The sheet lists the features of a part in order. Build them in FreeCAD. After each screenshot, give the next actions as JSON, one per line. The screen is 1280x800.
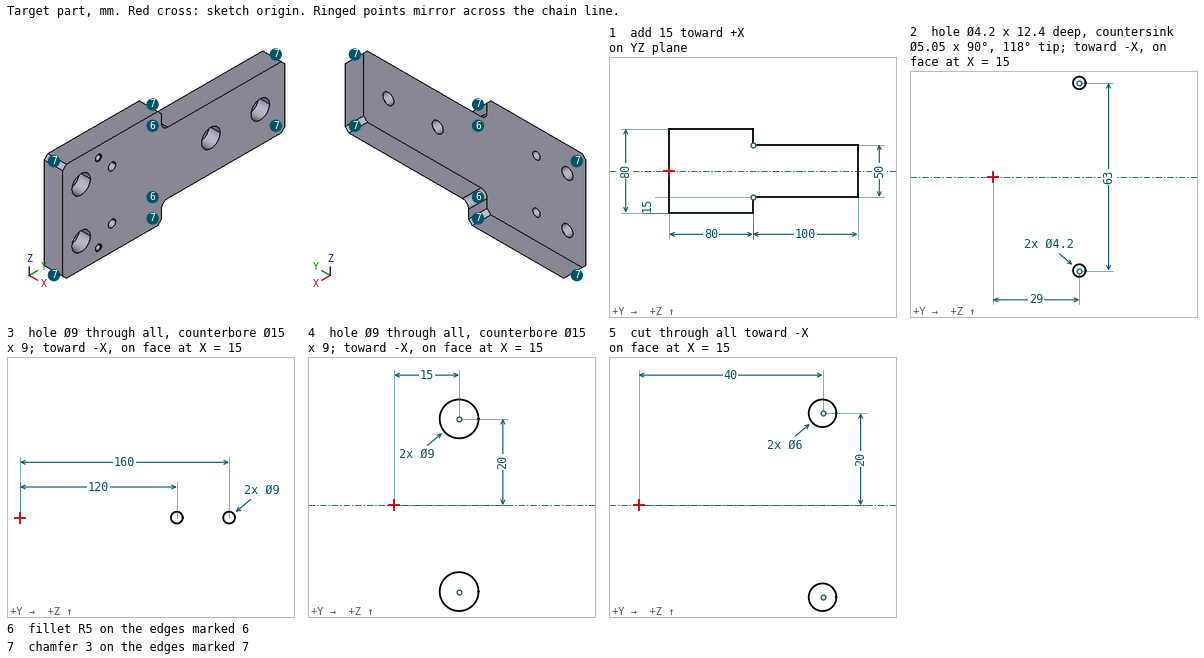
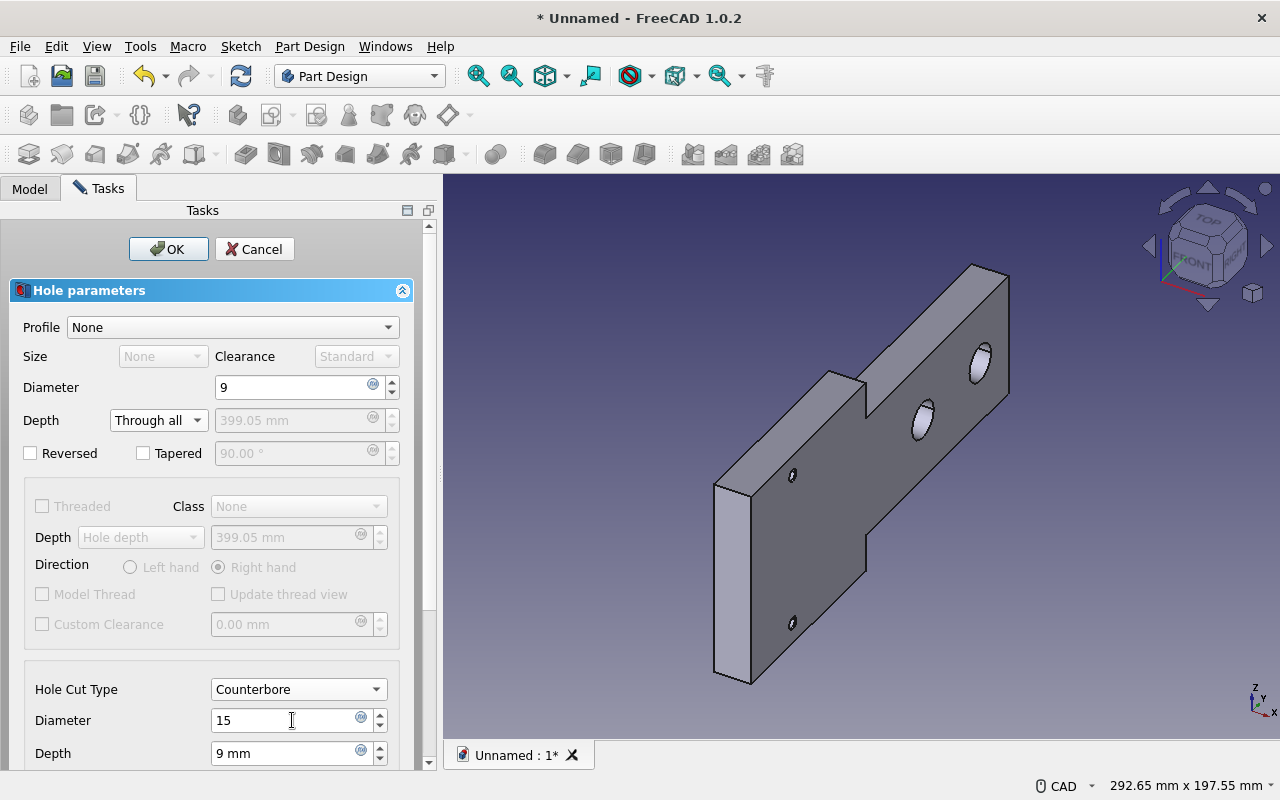
{"action": "left_click", "coordinate": [169, 249]}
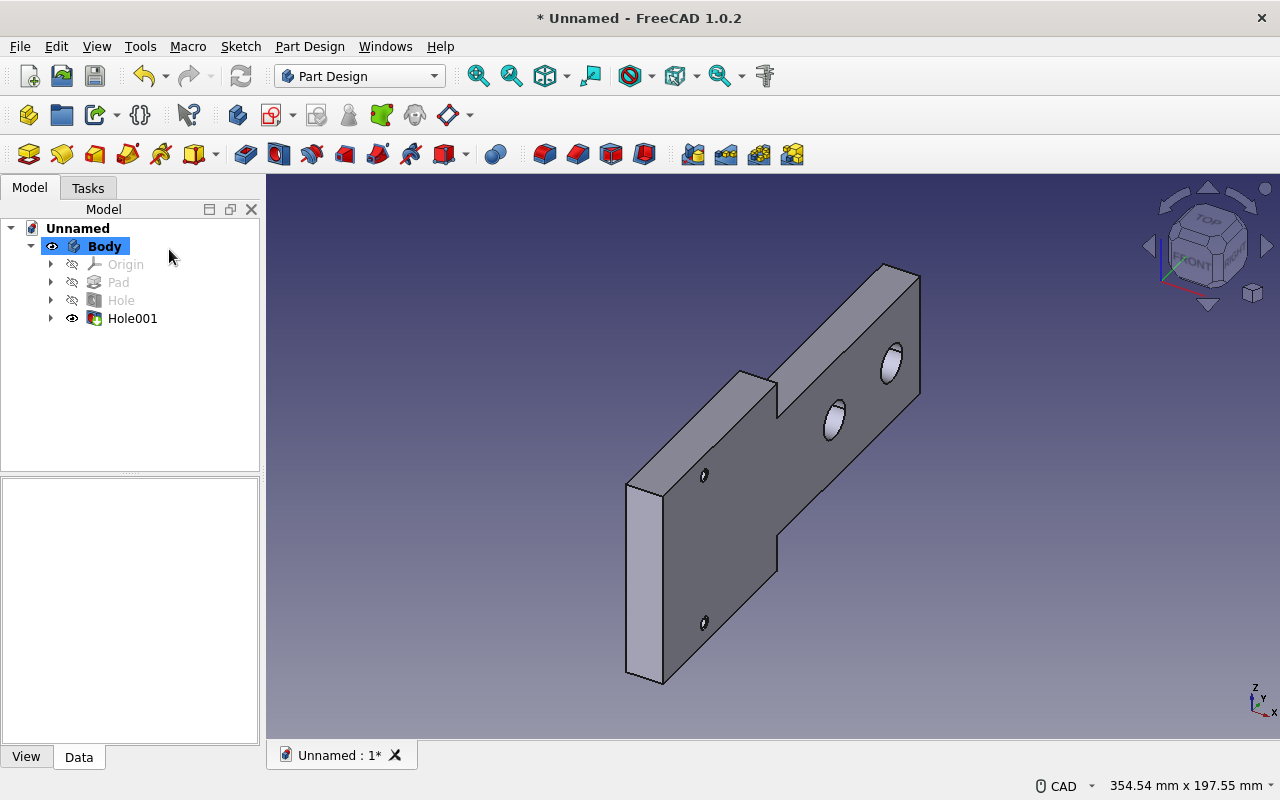
{"action": "left_click", "coordinate": [718, 535]}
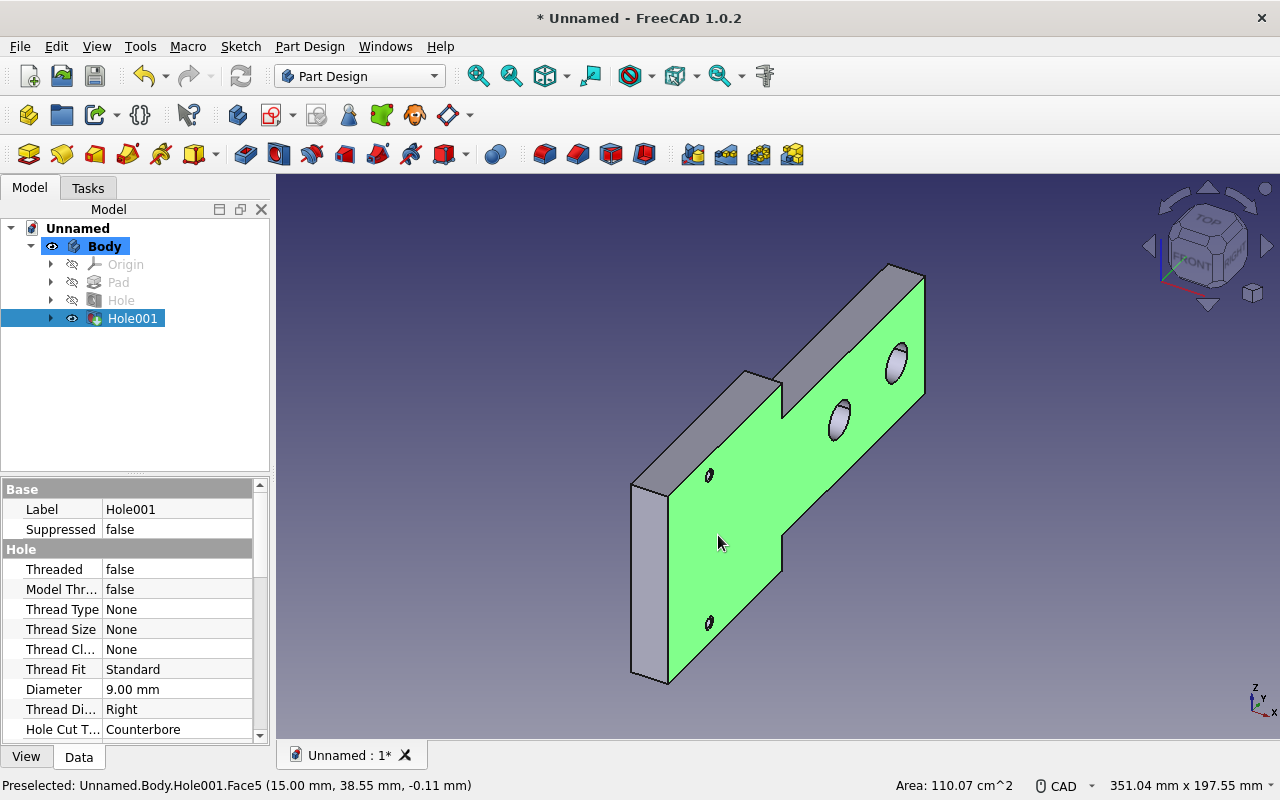
{"action": "left_click", "coordinate": [270, 116]}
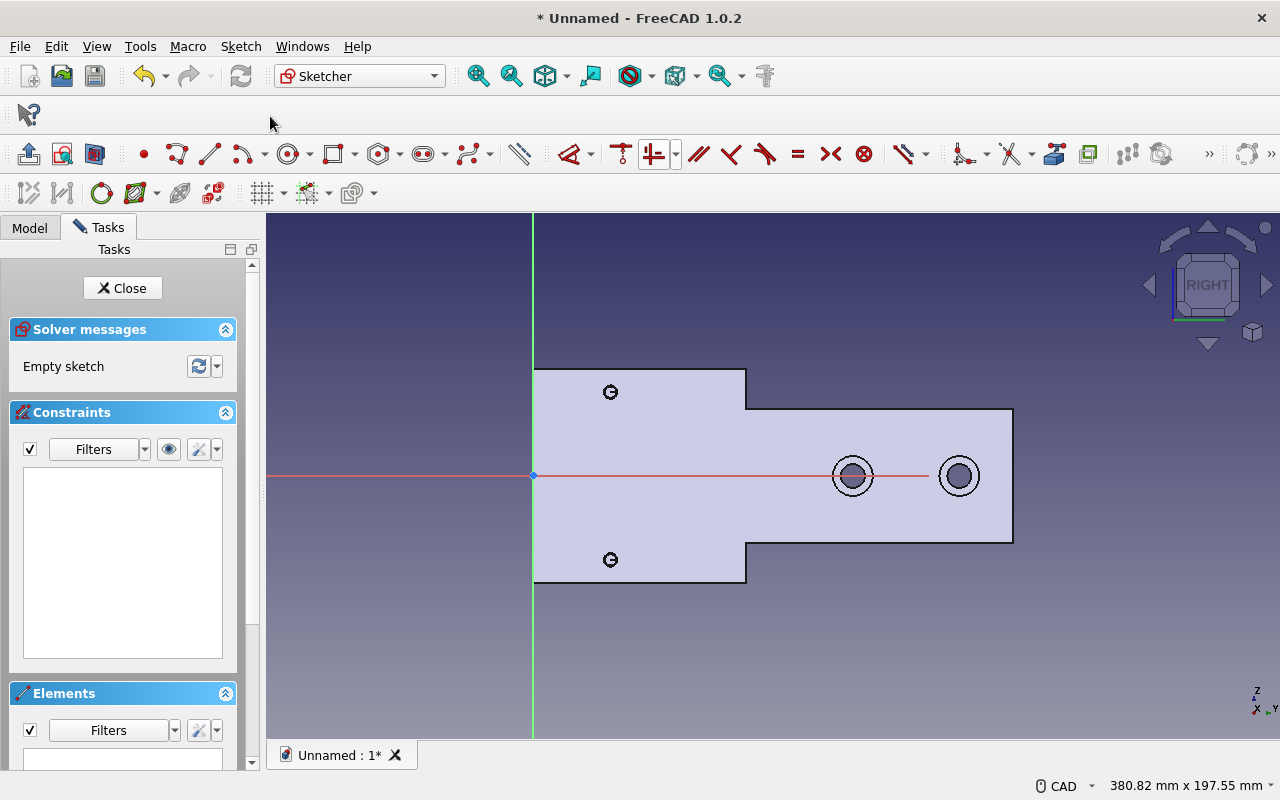
{"action": "scroll", "coordinate": [475, 476], "scroll_direction": "up", "scroll_amount": 5}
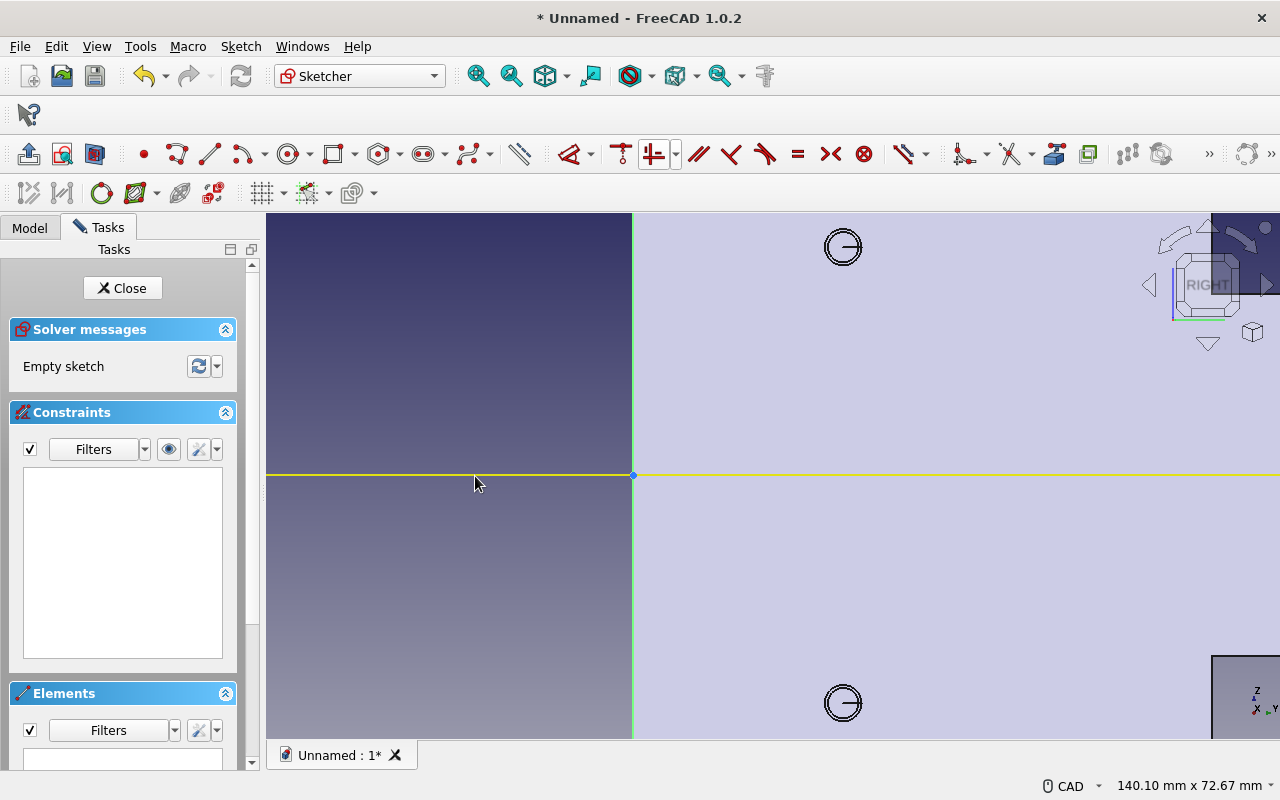
{"action": "left_click", "coordinate": [288, 154]}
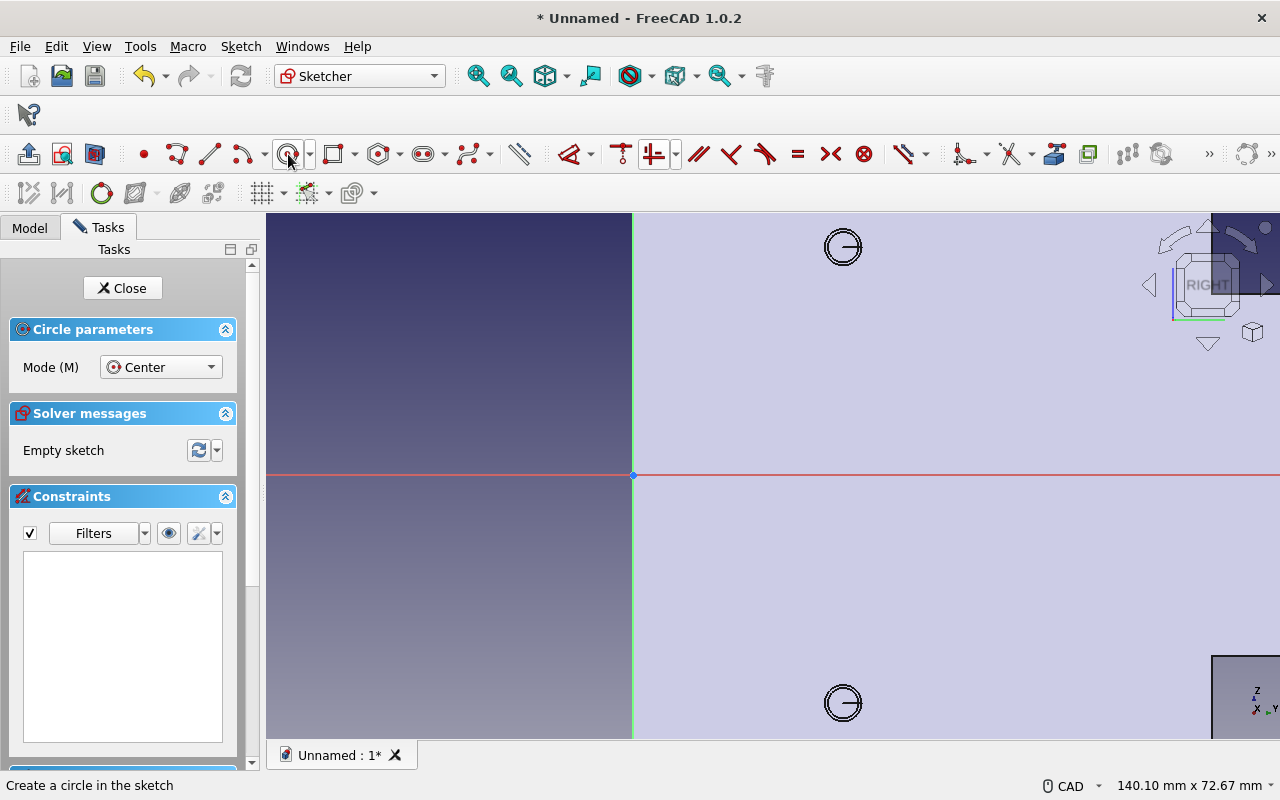
{"action": "left_click", "coordinate": [742, 330]}
{"action": "mouse_move", "coordinate": [765, 307]}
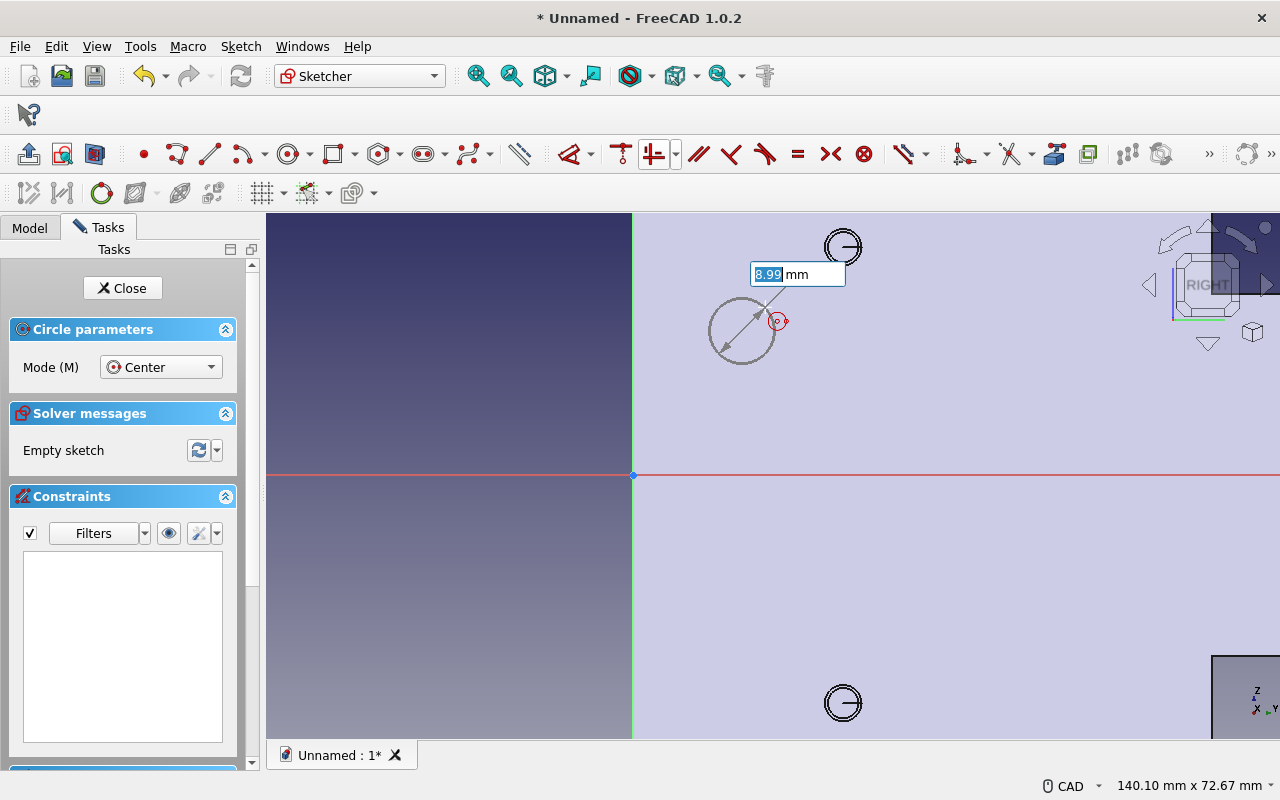
{"action": "type", "text": "9"}
{"action": "key", "text": "Return"}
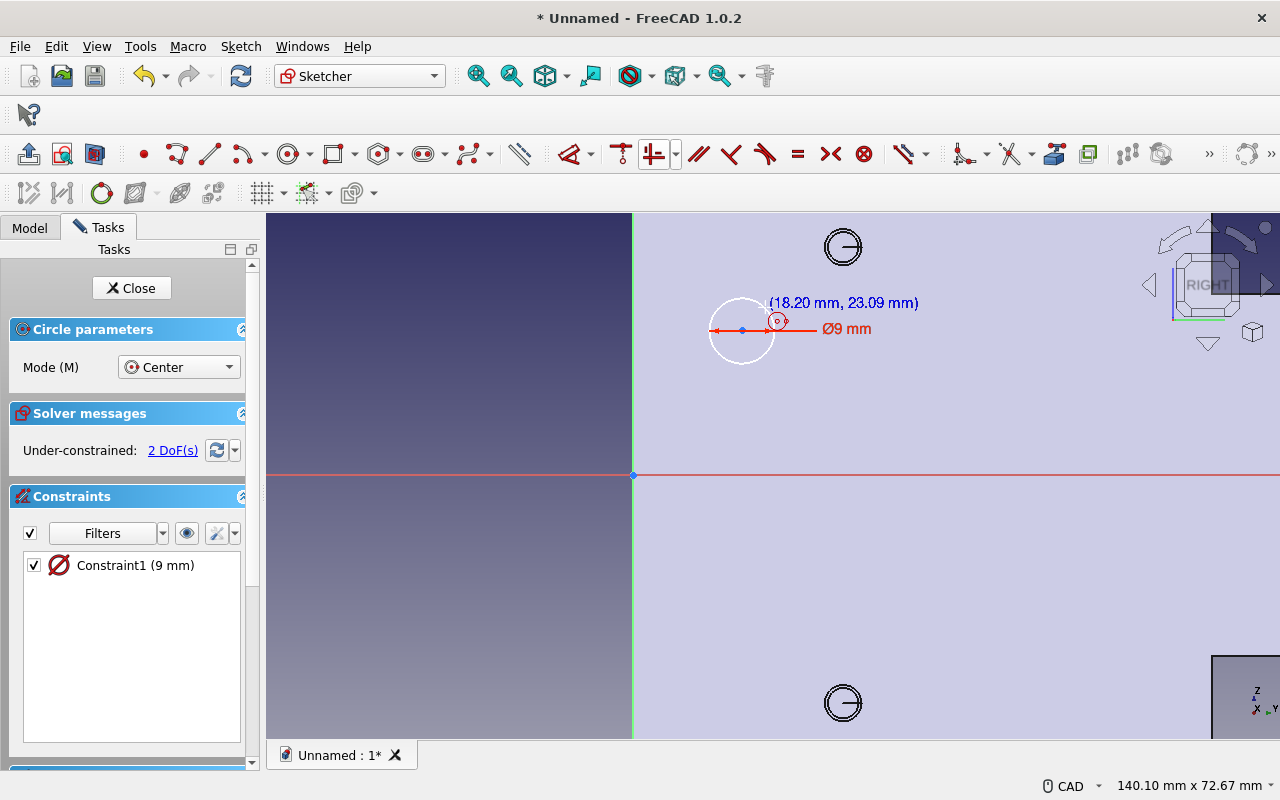
{"action": "left_click", "coordinate": [742, 620]}
{"action": "mouse_move", "coordinate": [765, 597]}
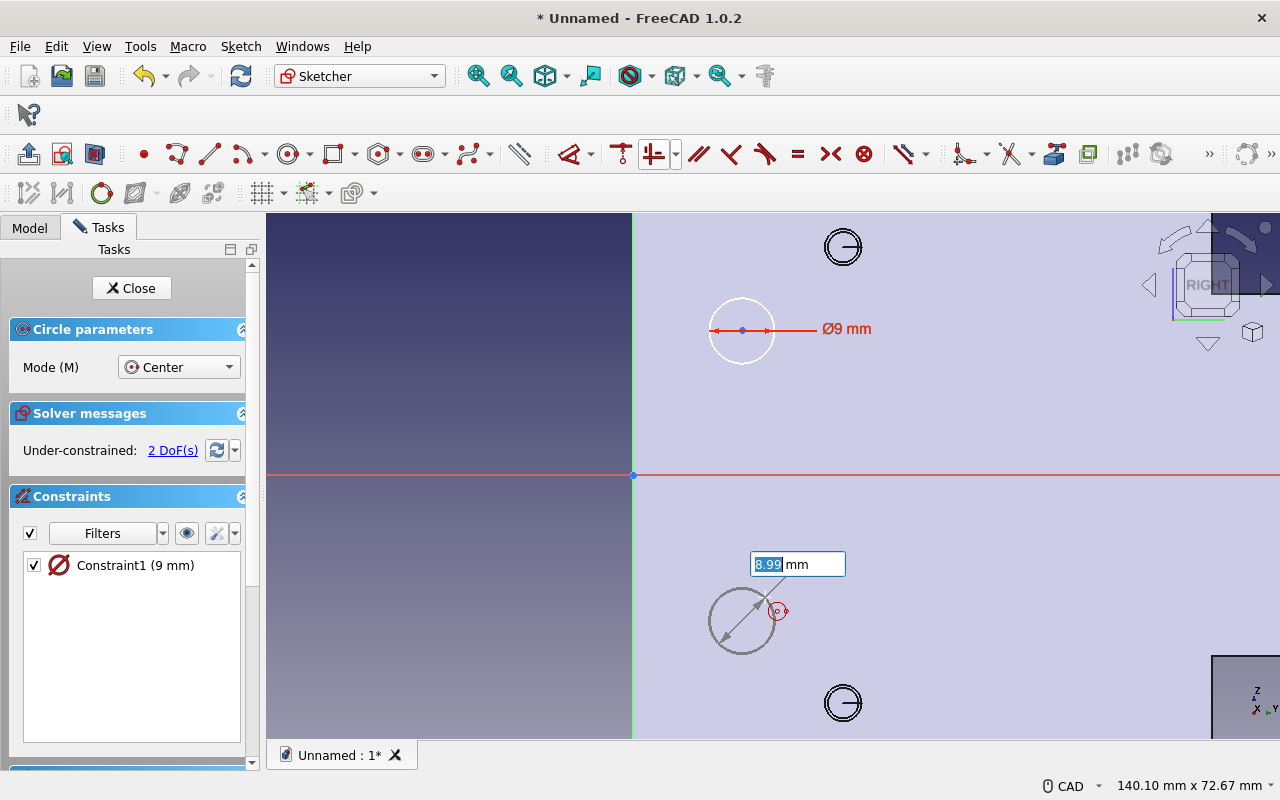
{"action": "type", "text": "9"}
{"action": "key", "text": "Return"}
{"action": "key", "text": "Escape"}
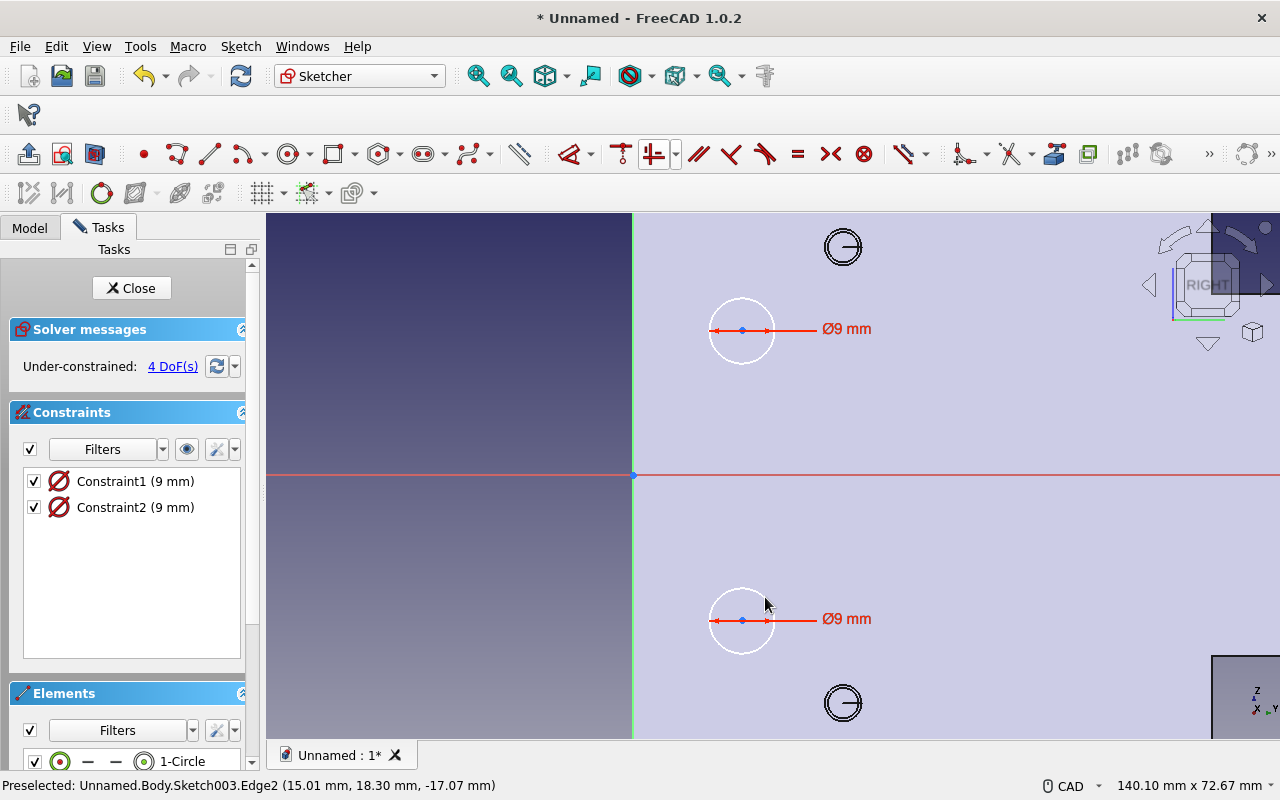
{"action": "left_click", "coordinate": [742, 331]}